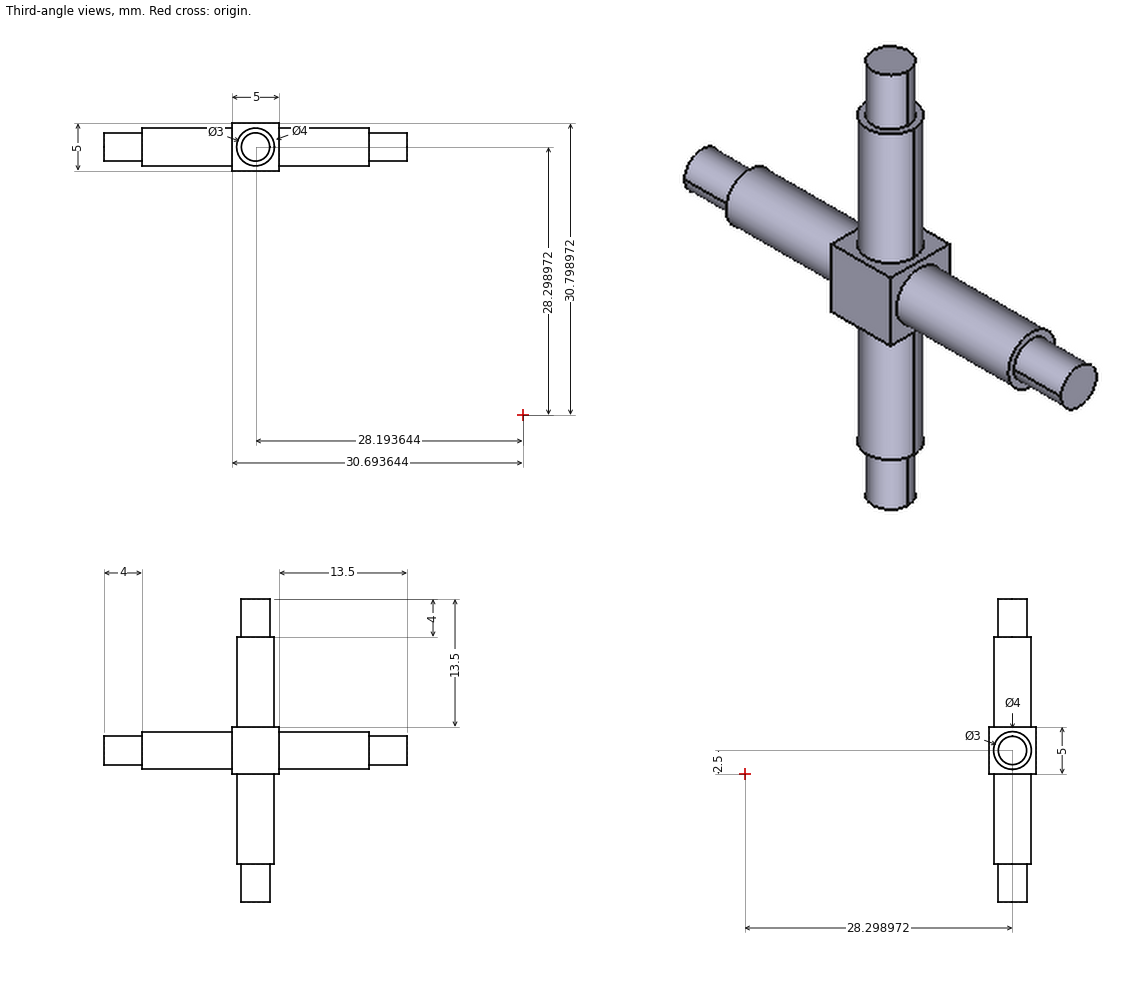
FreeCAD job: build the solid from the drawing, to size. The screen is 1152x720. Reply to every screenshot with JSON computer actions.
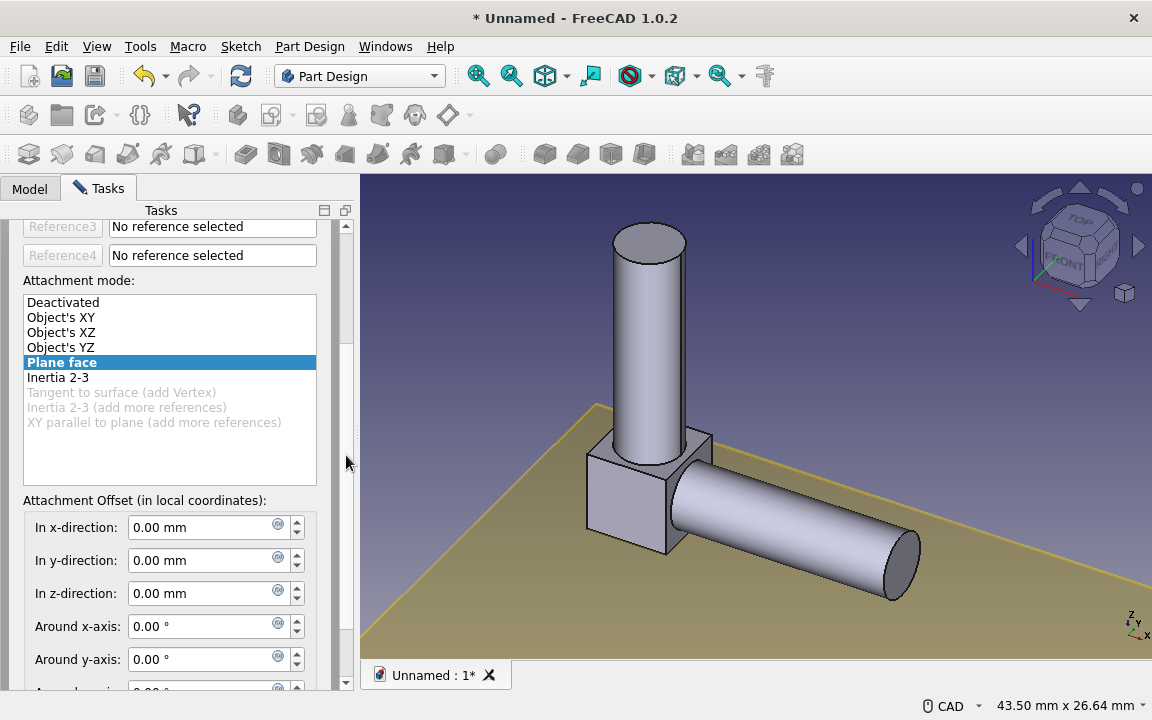
{"action": "triple_click", "coordinate": [210, 594]}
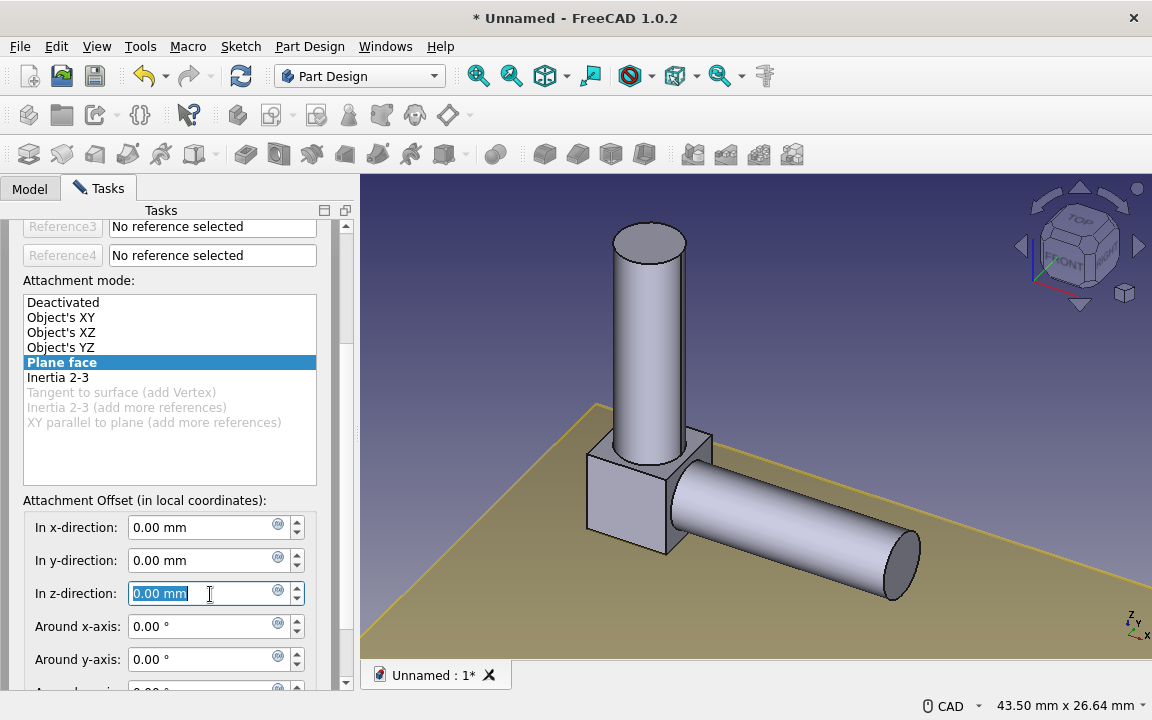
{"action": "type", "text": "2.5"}
{"action": "key", "text": "Tab"}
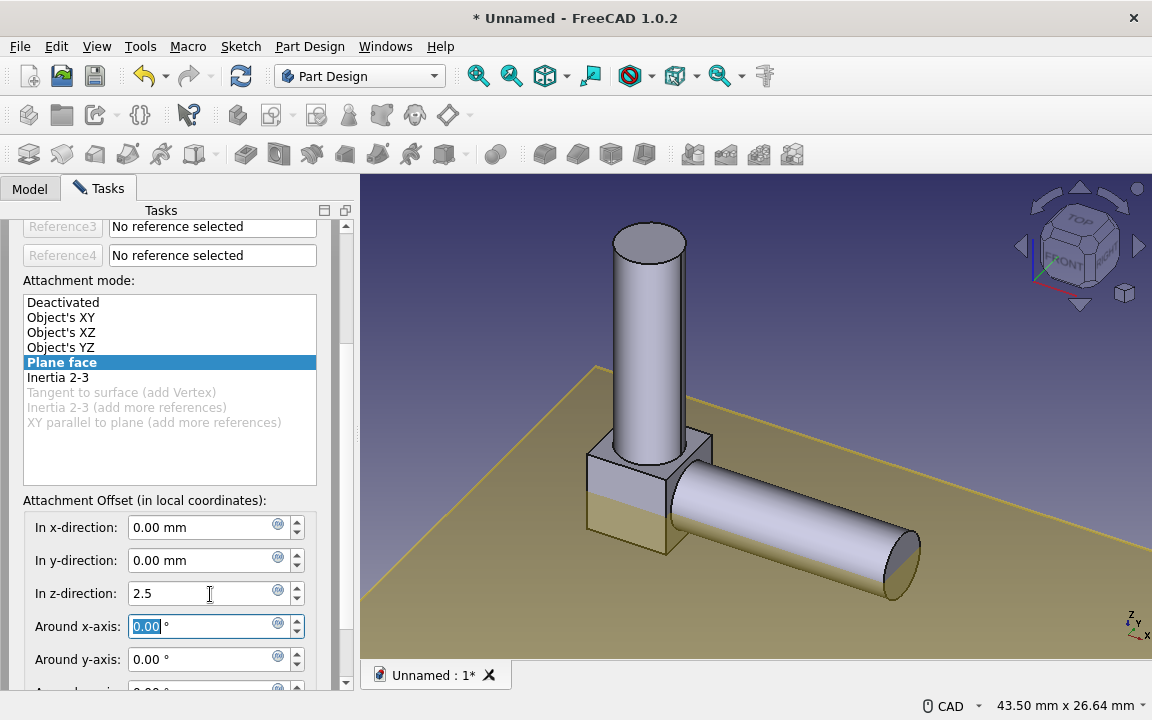
{"action": "scroll", "coordinate": [346, 455], "scroll_direction": "up", "scroll_amount": 4}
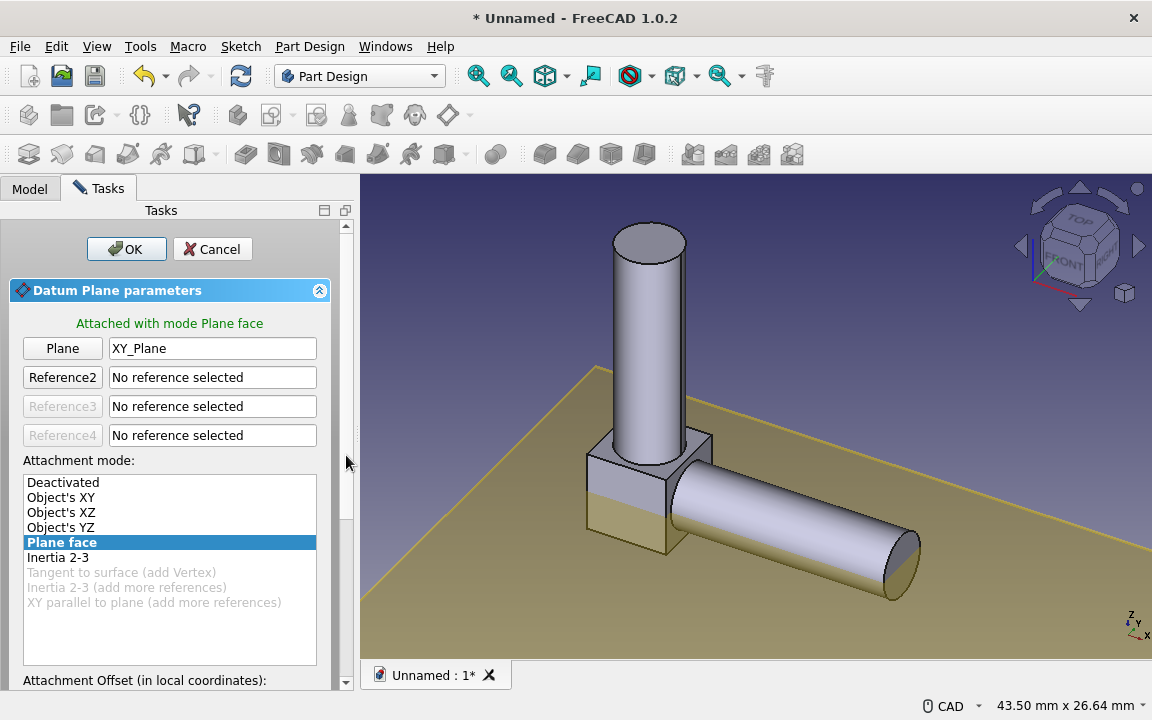
{"action": "left_click", "coordinate": [127, 249]}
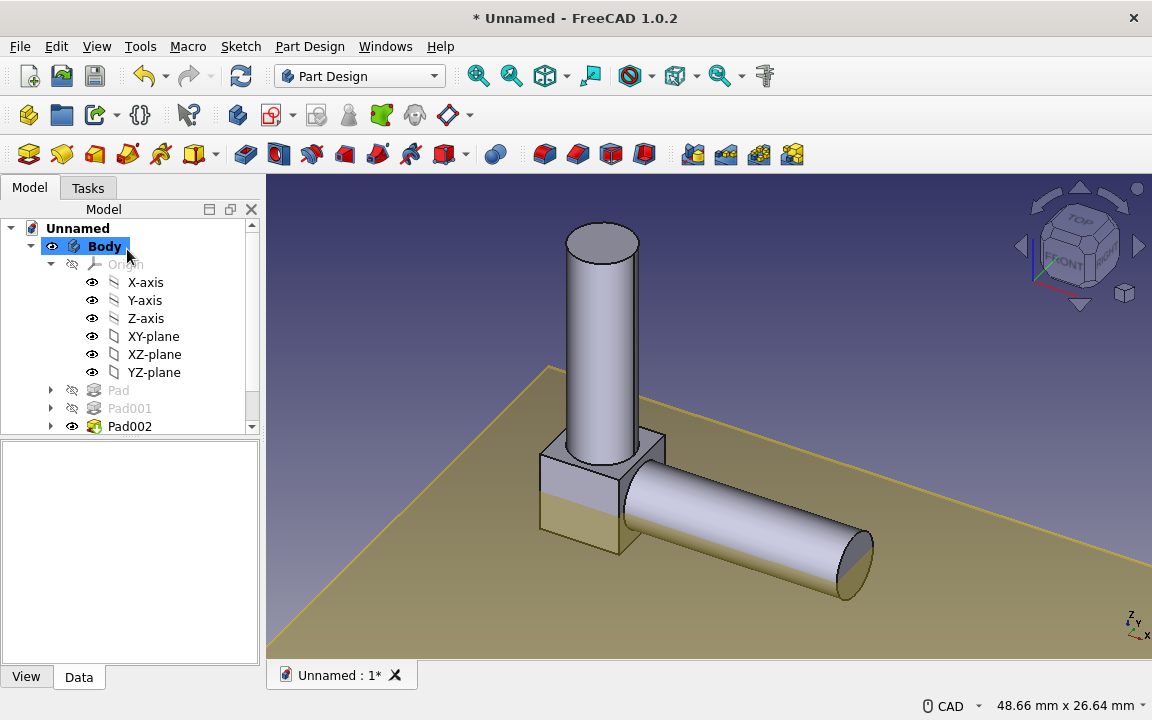
{"action": "left_click", "coordinate": [117, 408]}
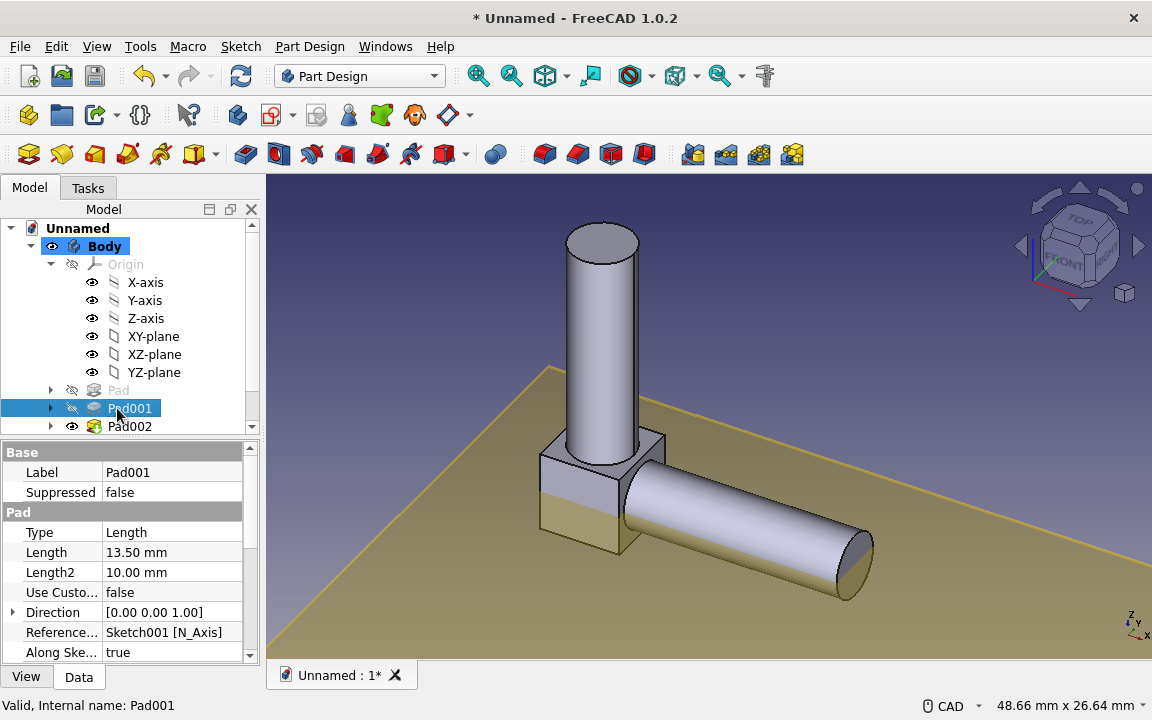
{"action": "left_click", "coordinate": [693, 154]}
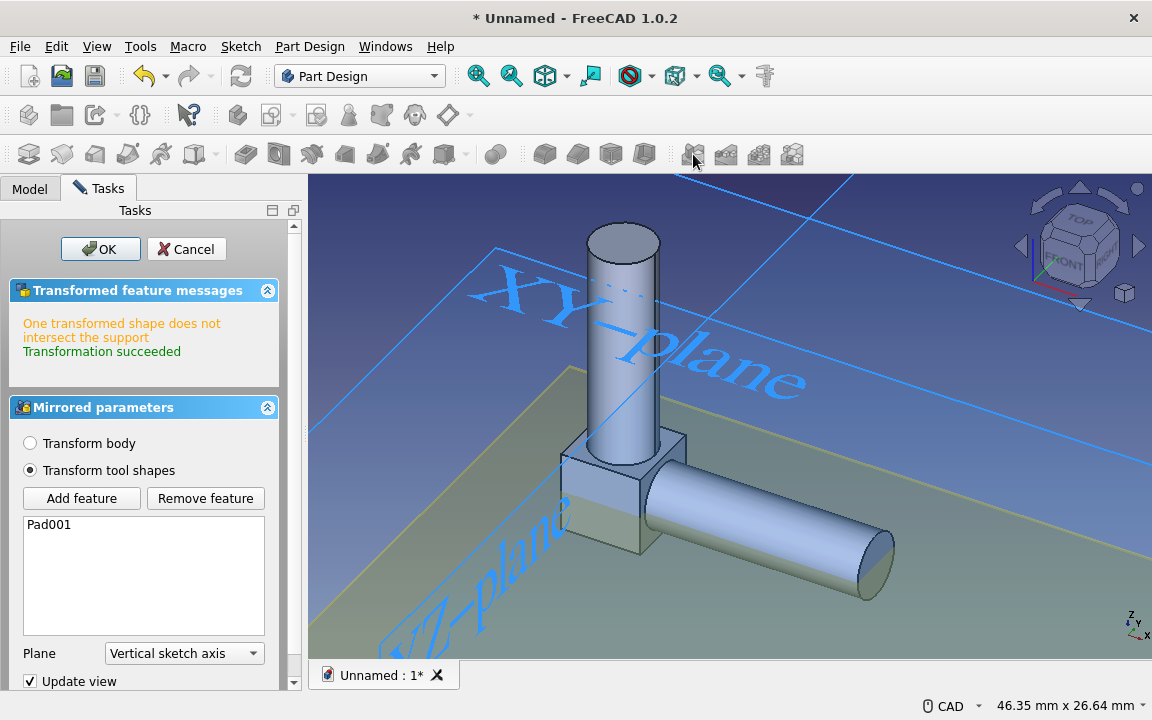
{"action": "left_click", "coordinate": [185, 654]}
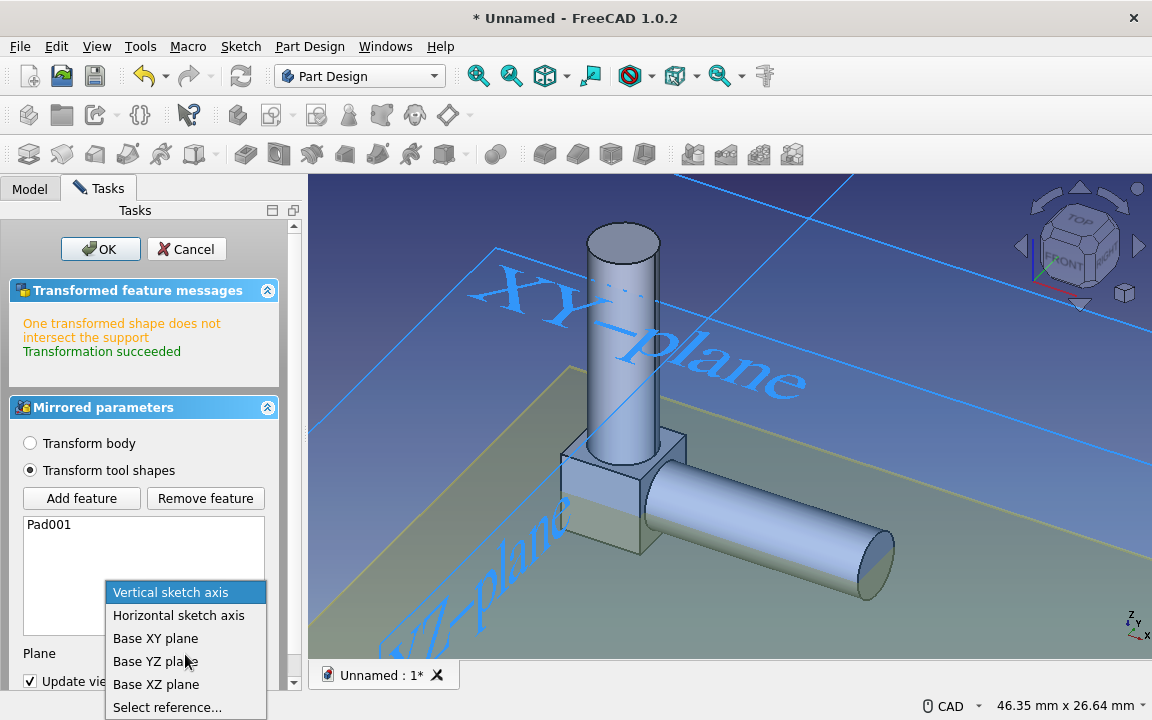
{"action": "left_click", "coordinate": [184, 708]}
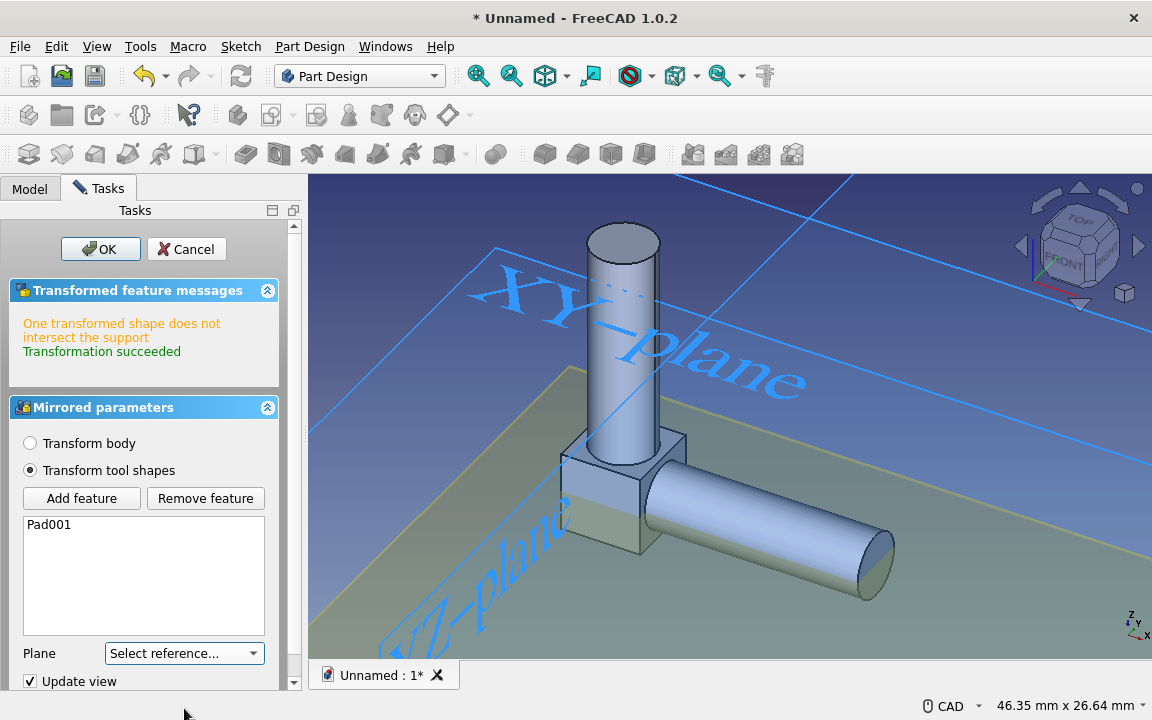
{"action": "left_click", "coordinate": [30, 188]}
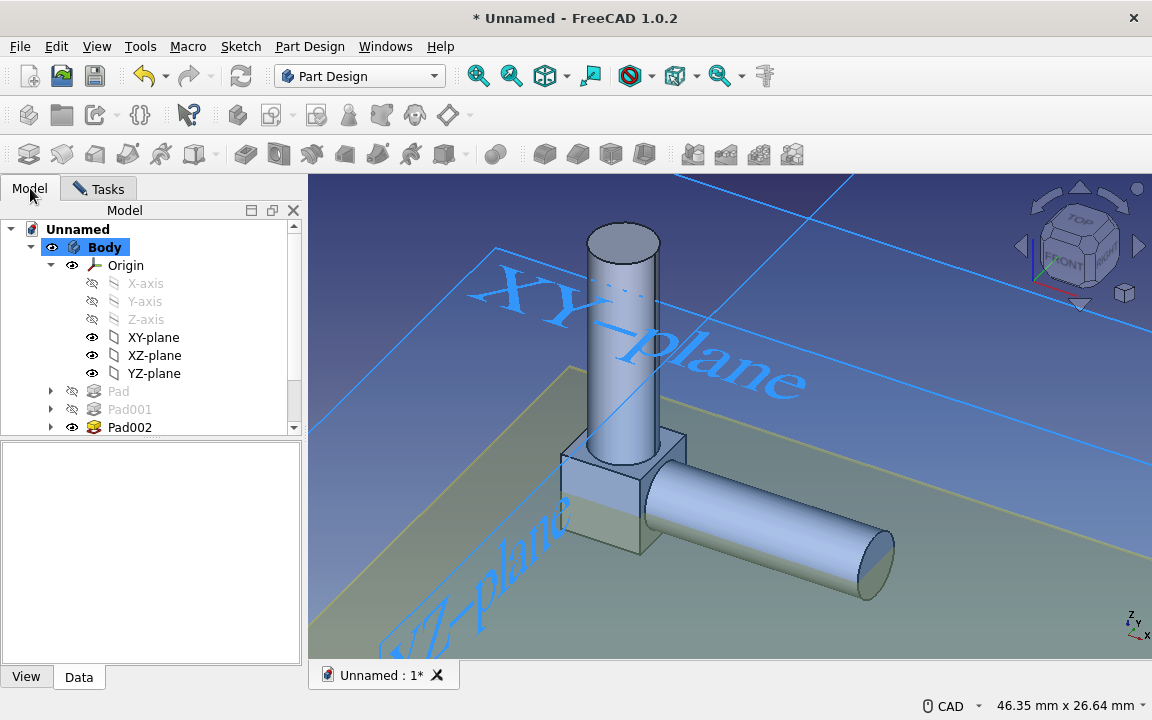
{"action": "scroll", "coordinate": [101, 333], "scroll_direction": "down", "scroll_amount": 3}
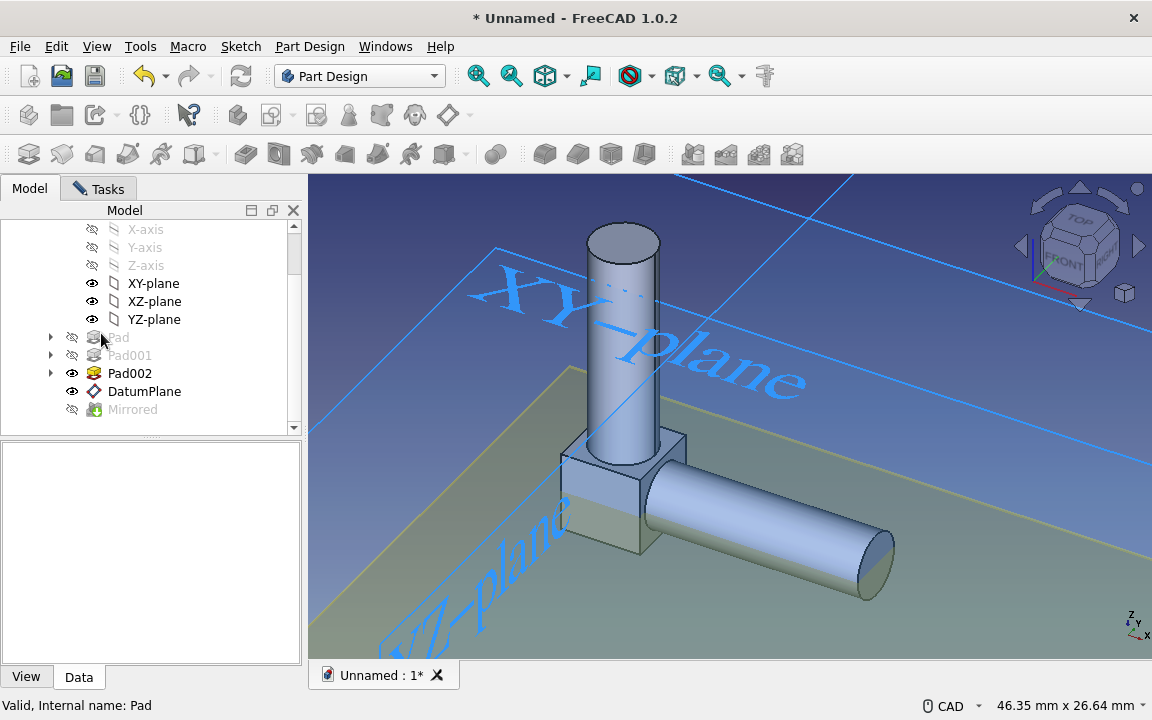
{"action": "left_click", "coordinate": [117, 391]}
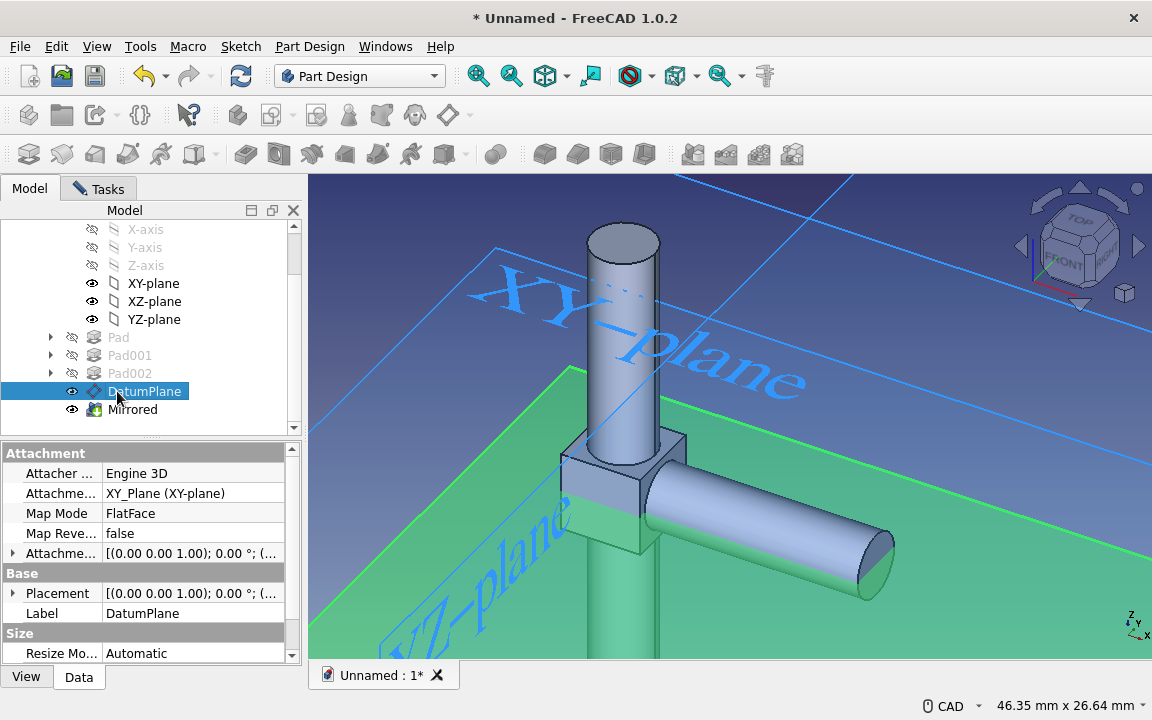
{"action": "left_click", "coordinate": [98, 188]}